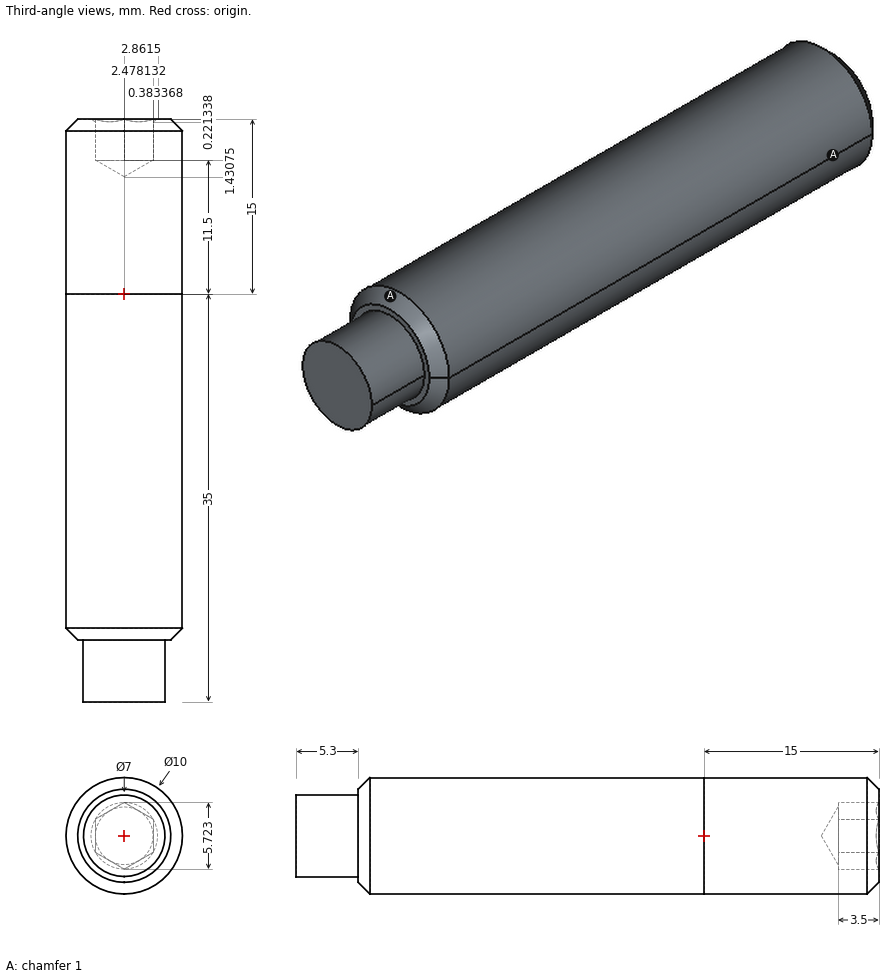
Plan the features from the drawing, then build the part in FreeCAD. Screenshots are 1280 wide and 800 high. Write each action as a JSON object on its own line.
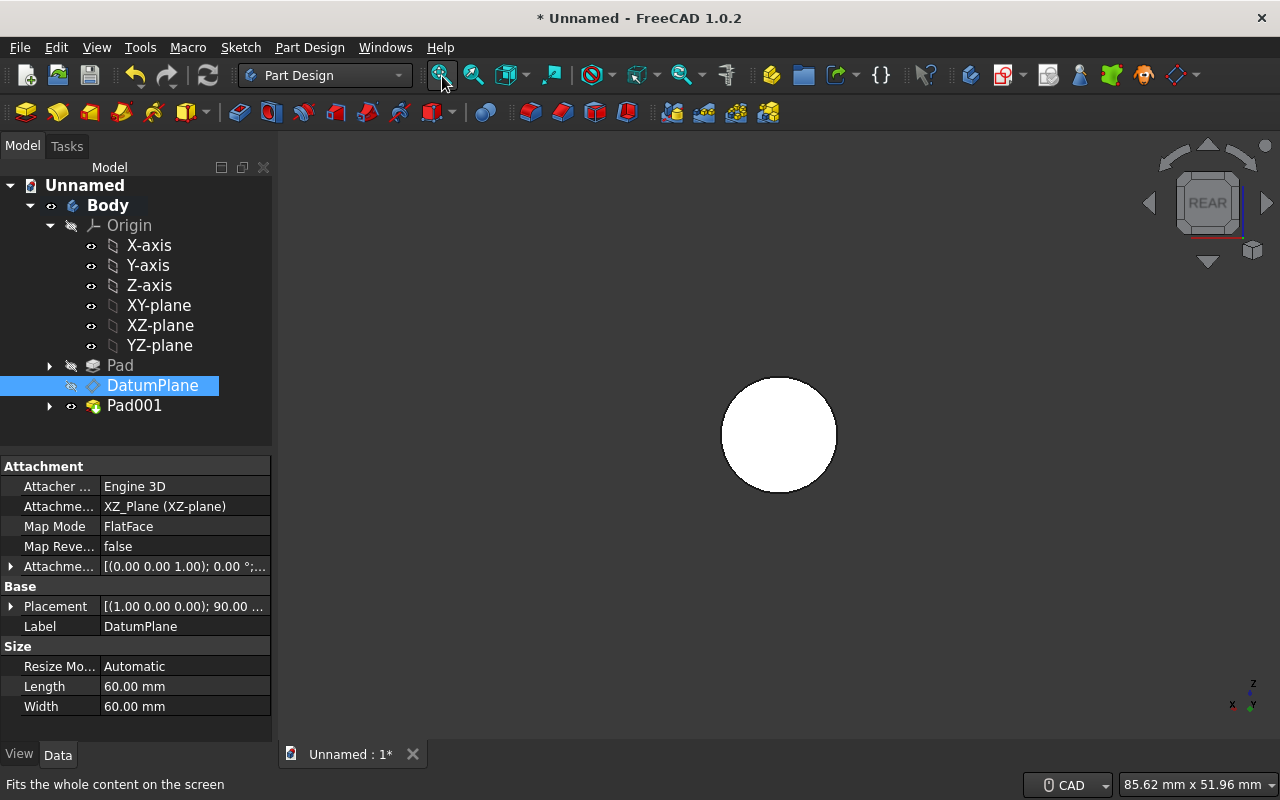
{"action": "left_click", "coordinate": [779, 434]}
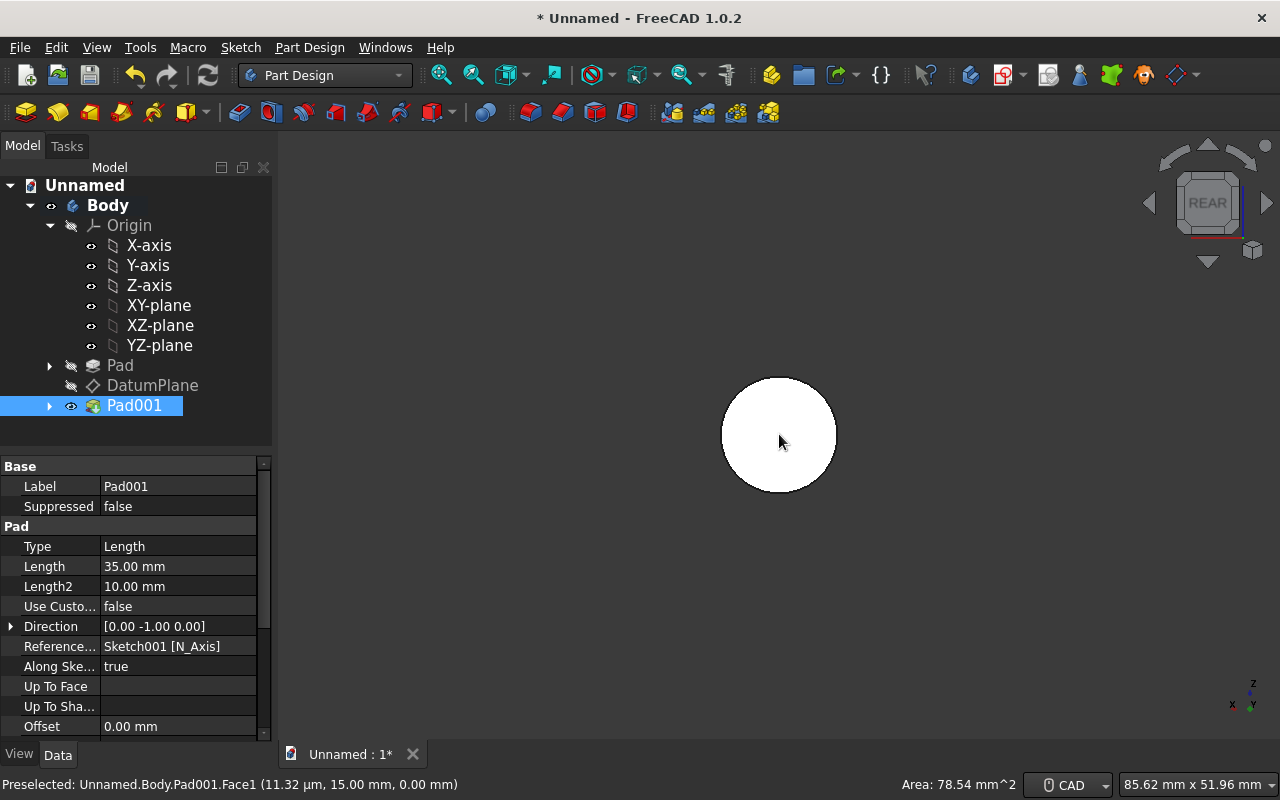
{"action": "left_click", "coordinate": [1004, 76]}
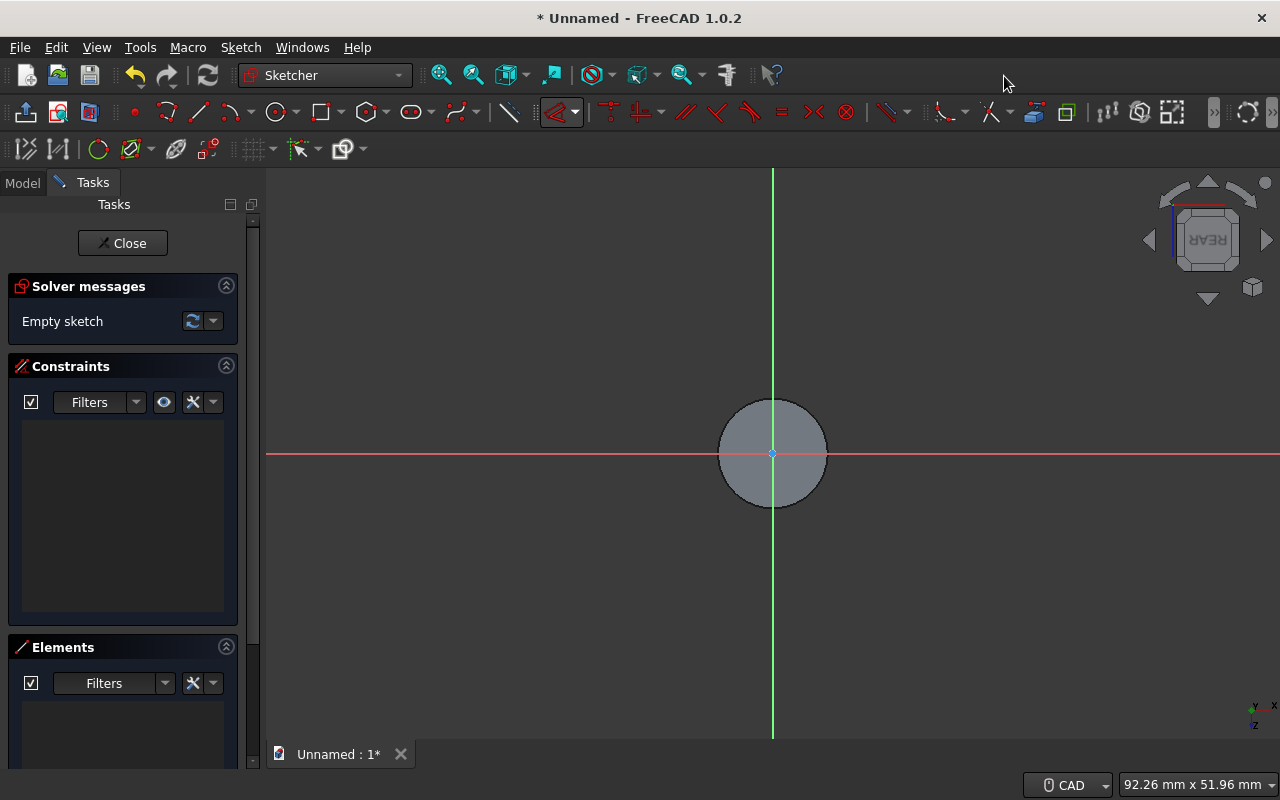
{"action": "scroll", "coordinate": [786, 453], "scroll_direction": "up", "scroll_amount": 9}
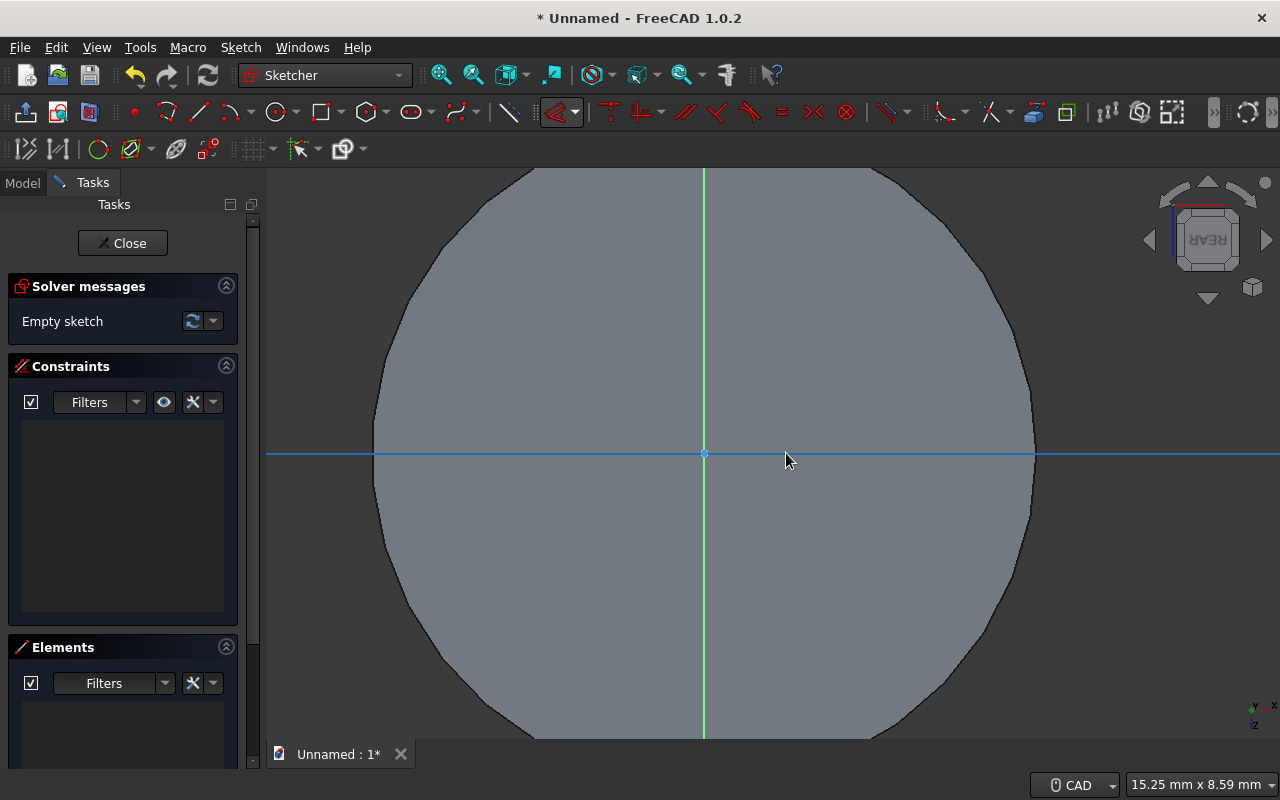
{"action": "left_click", "coordinate": [366, 112]}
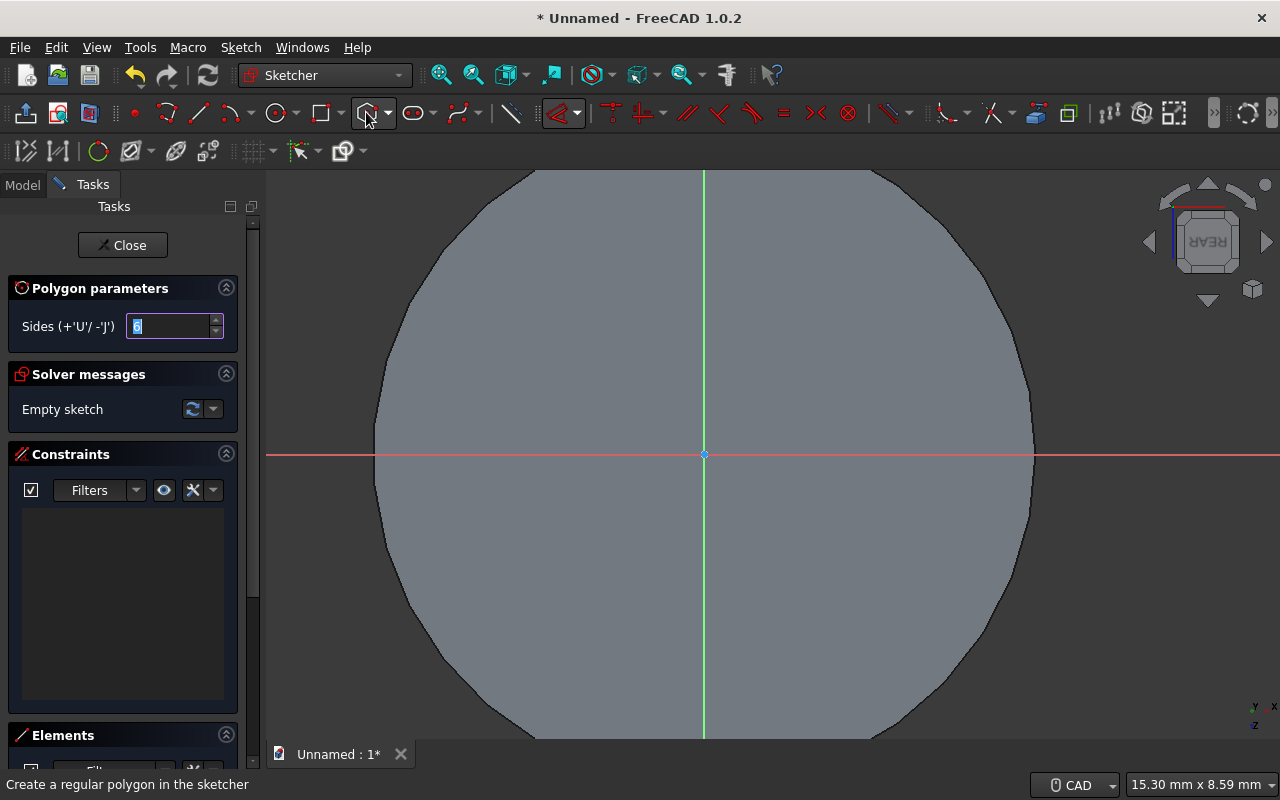
{"action": "left_click", "coordinate": [704, 454]}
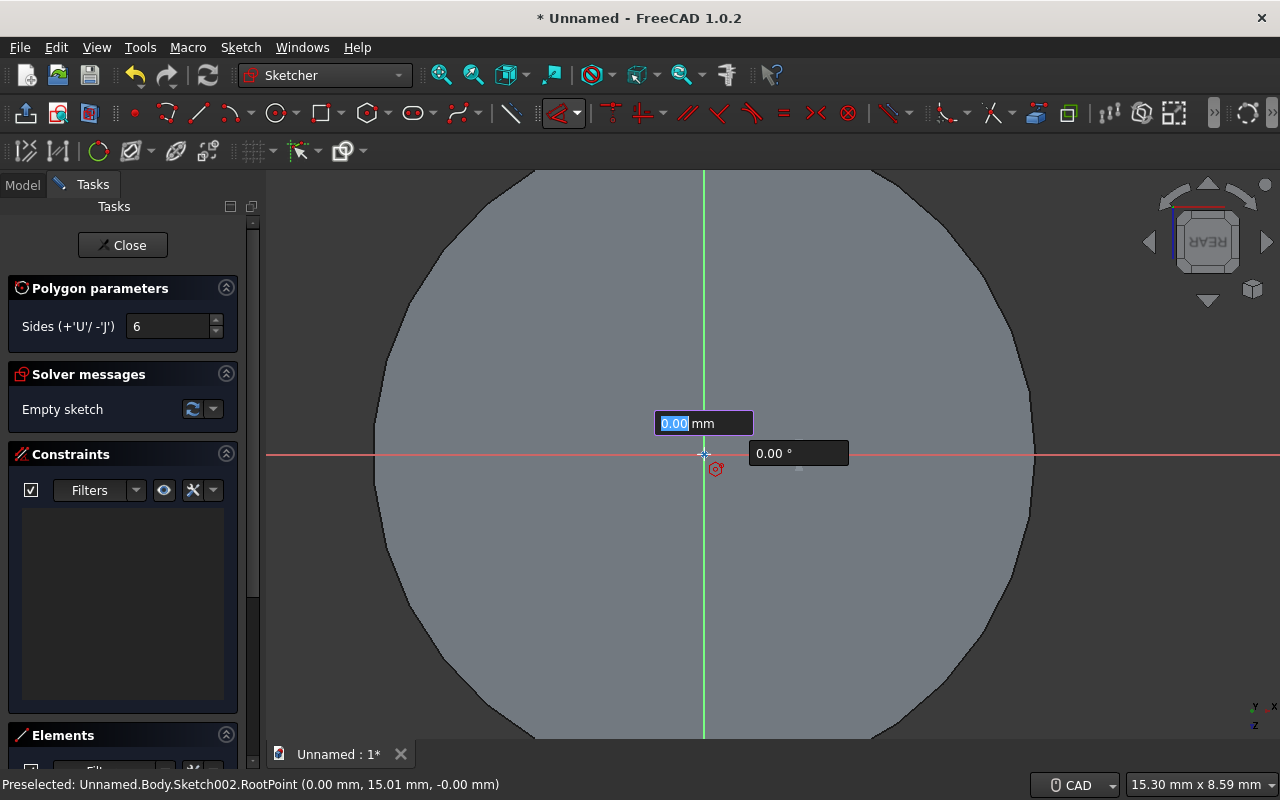
{"action": "left_click", "coordinate": [704, 265]}
{"action": "right_click", "coordinate": [704, 265]}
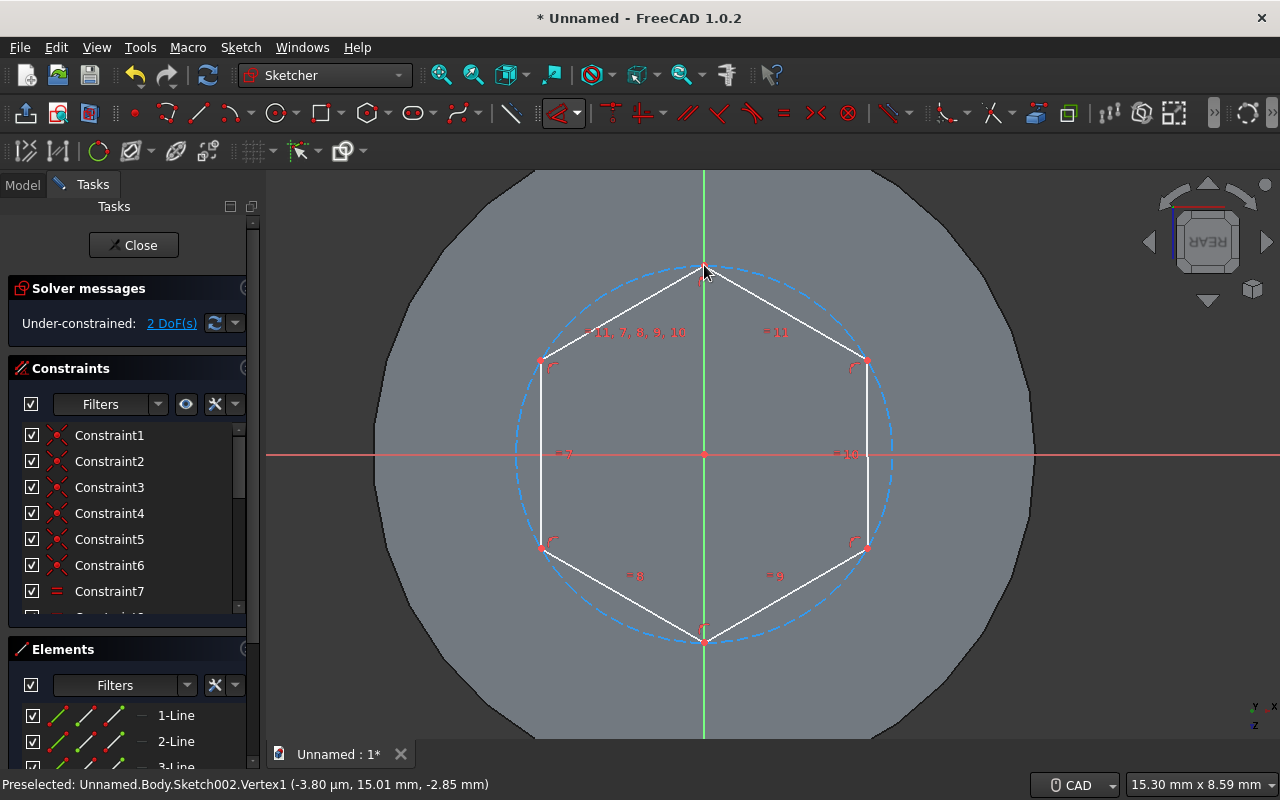
{"action": "left_click", "coordinate": [541, 417]}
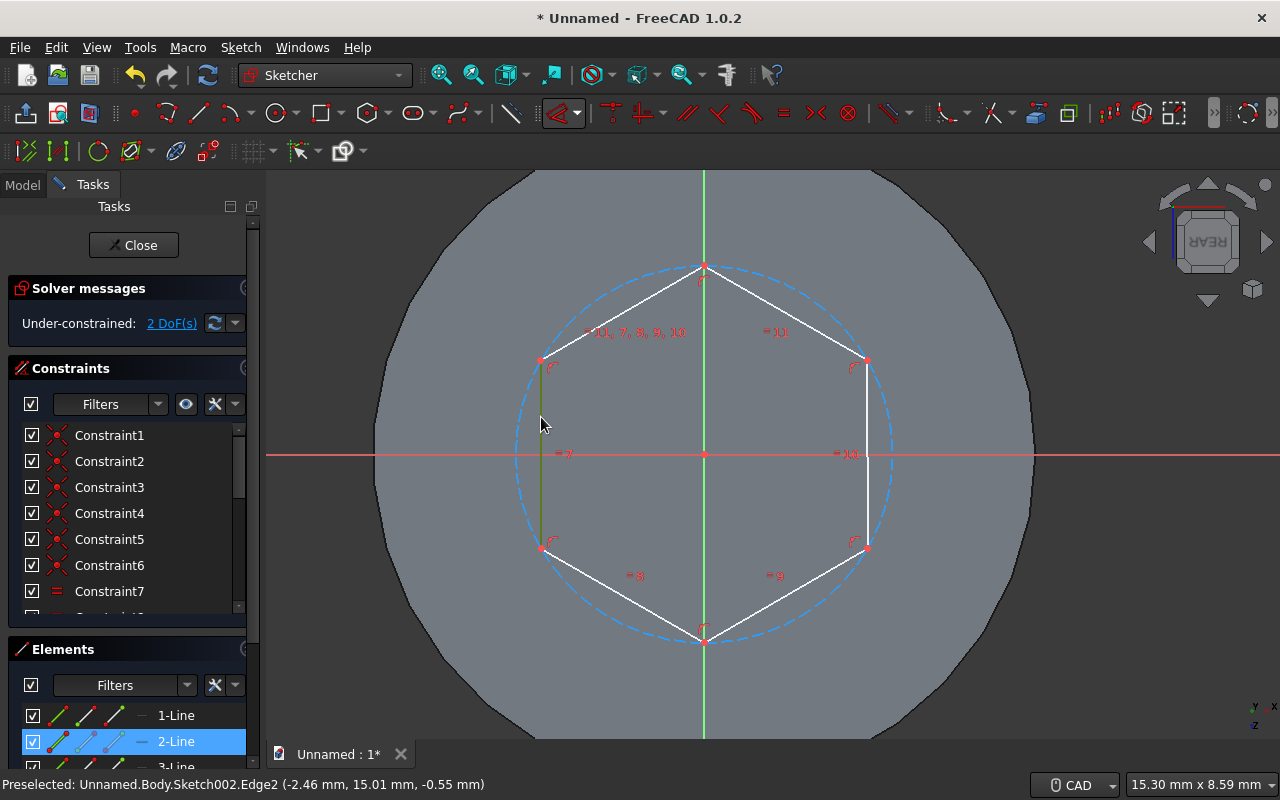
{"action": "key", "text": "v"}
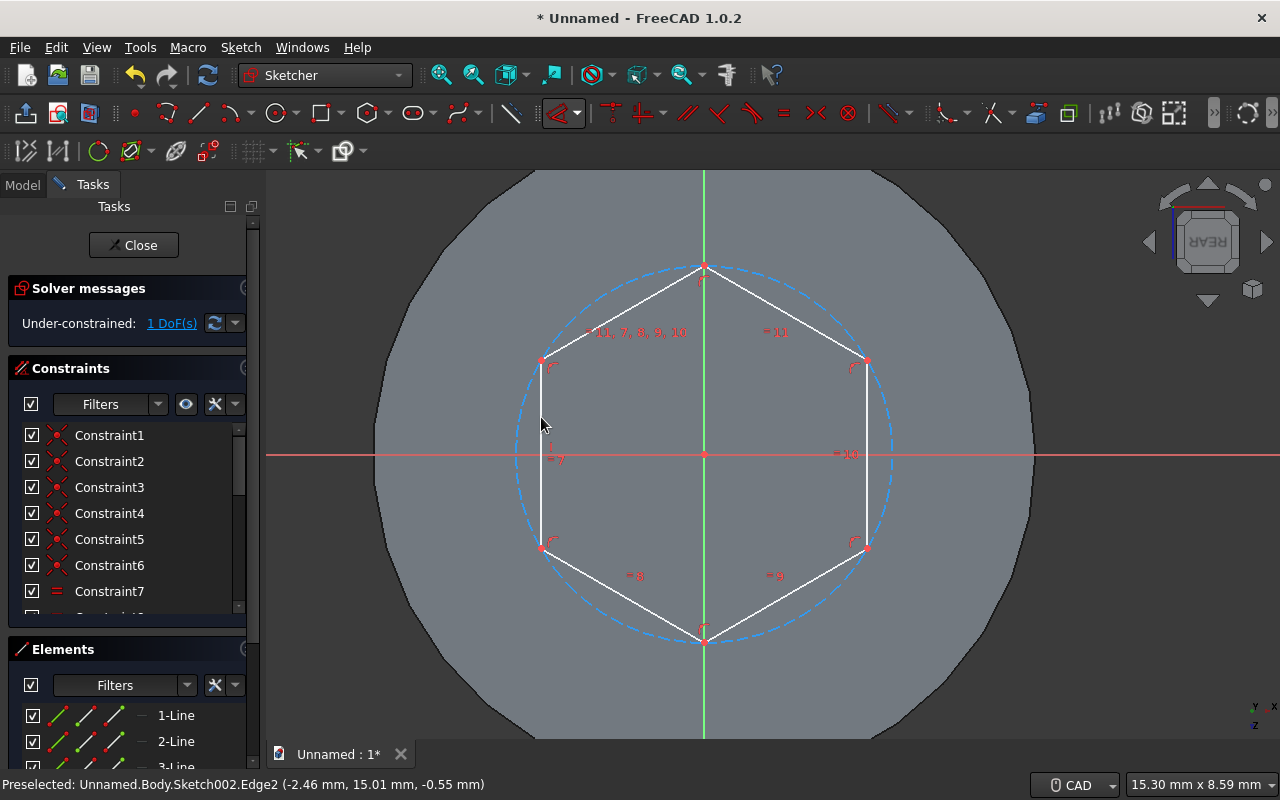
{"action": "left_click", "coordinate": [704, 643]}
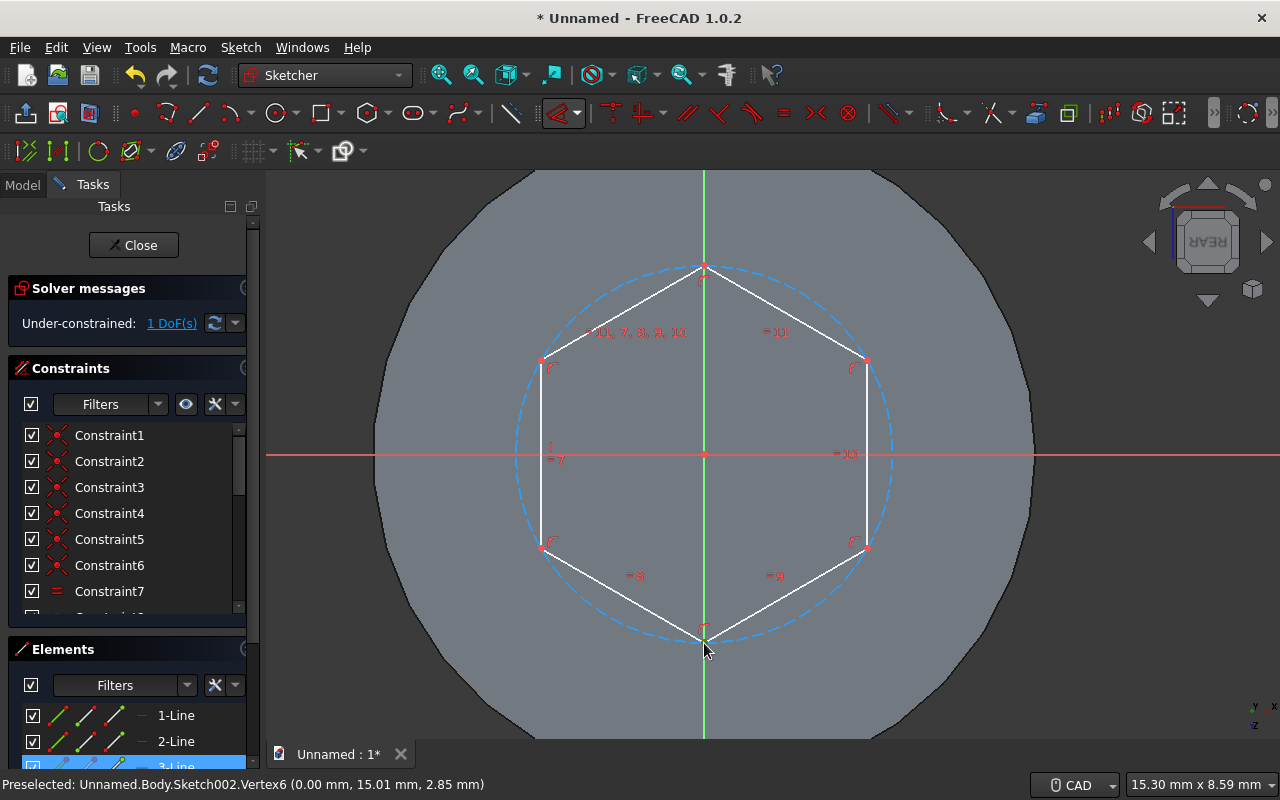
{"action": "left_click", "coordinate": [704, 266]}